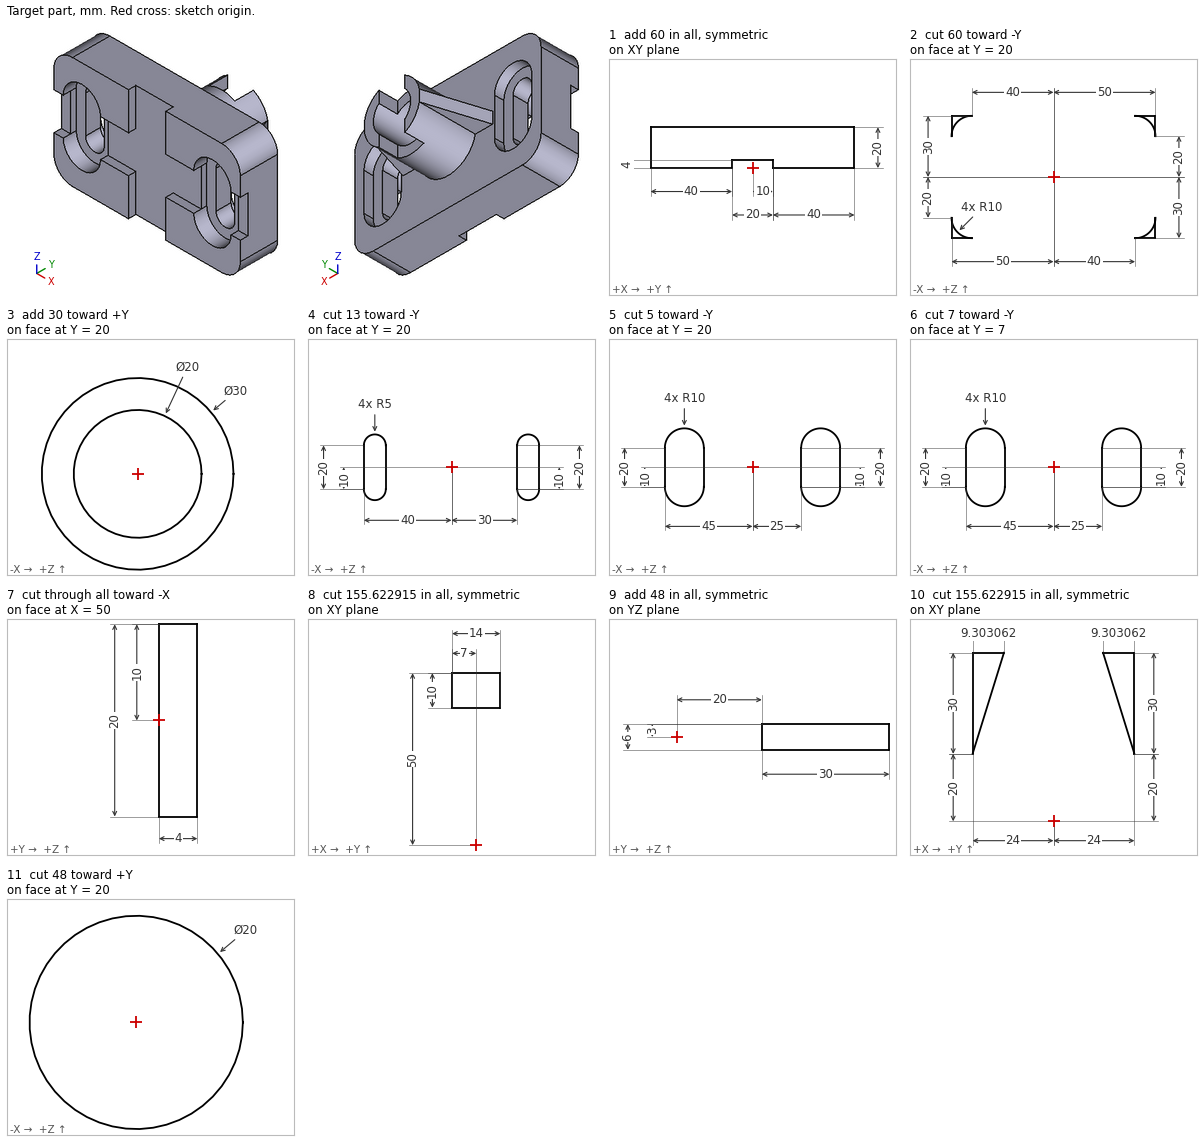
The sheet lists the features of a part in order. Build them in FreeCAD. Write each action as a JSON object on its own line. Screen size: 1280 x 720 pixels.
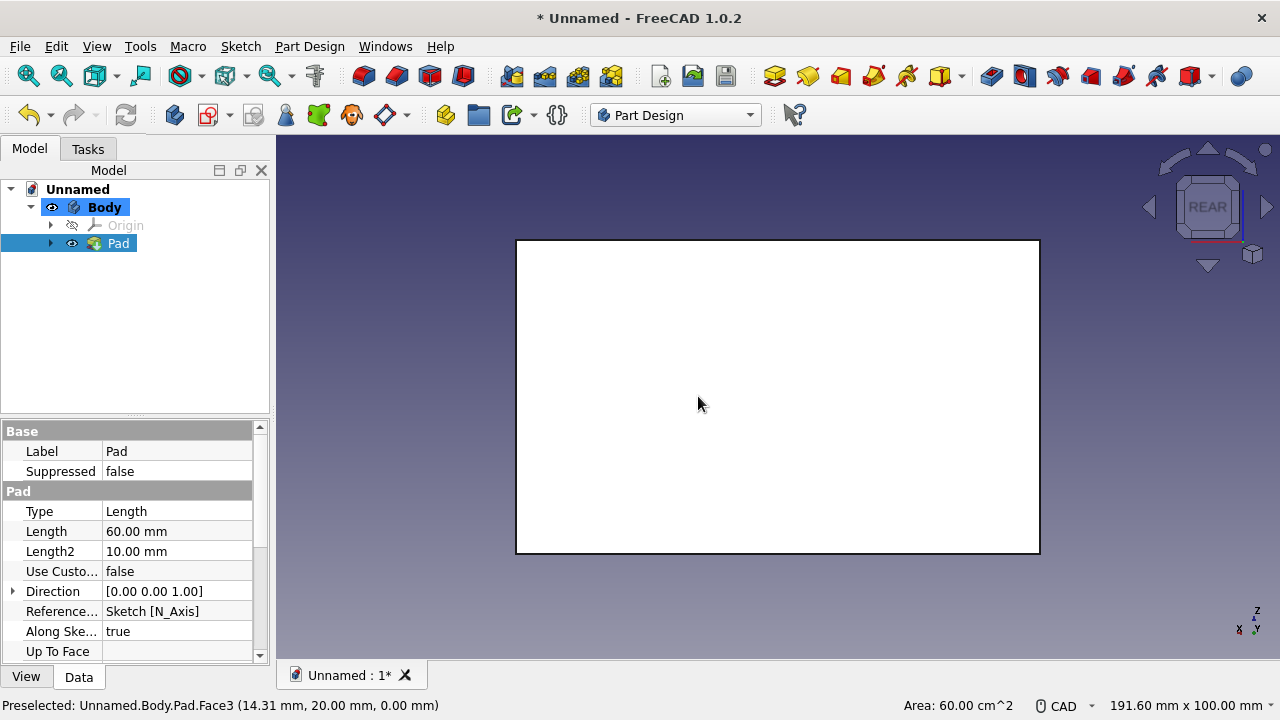
{"action": "left_click", "coordinate": [208, 116]}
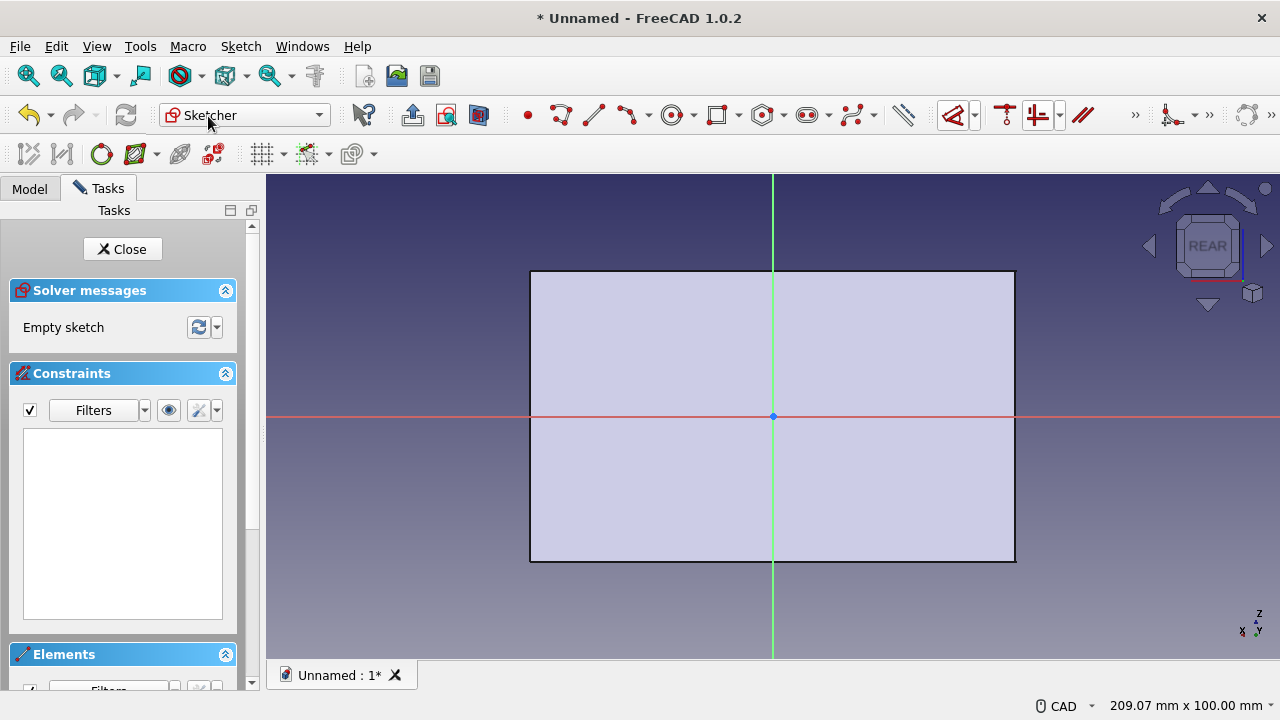
{"action": "left_click", "coordinate": [561, 116]}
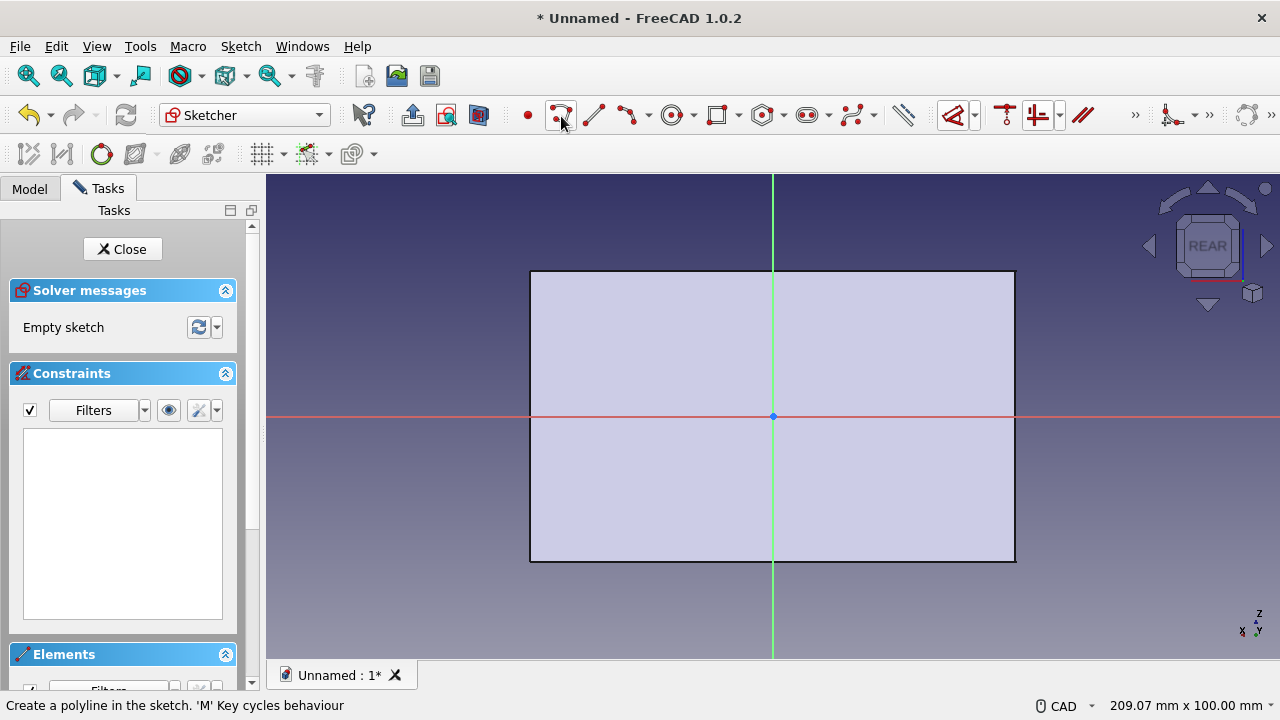
{"action": "left_click", "coordinate": [531, 513]}
{"action": "left_click", "coordinate": [531, 562]}
{"action": "left_click", "coordinate": [579, 562]}
{"action": "right_click", "coordinate": [579, 562]}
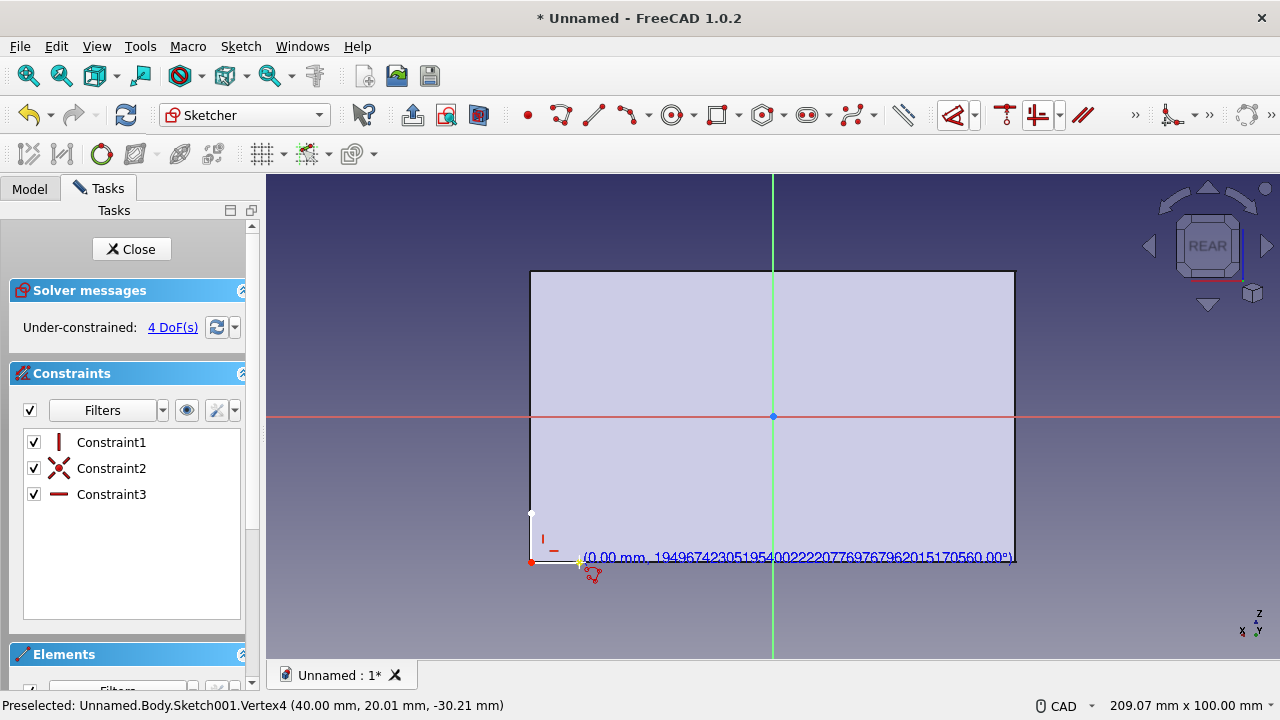
{"action": "key", "text": "g 3 a"}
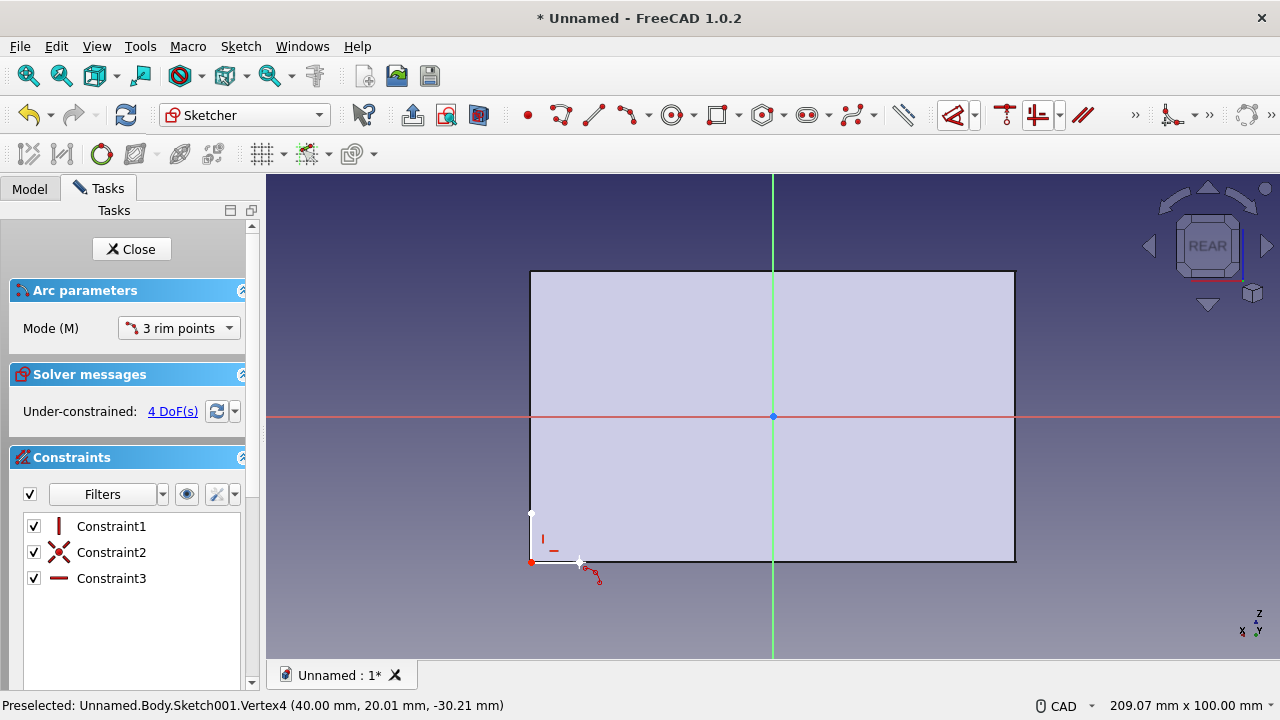
{"action": "left_click", "coordinate": [579, 563]}
{"action": "left_click", "coordinate": [531, 514]}
{"action": "left_click", "coordinate": [545, 548]}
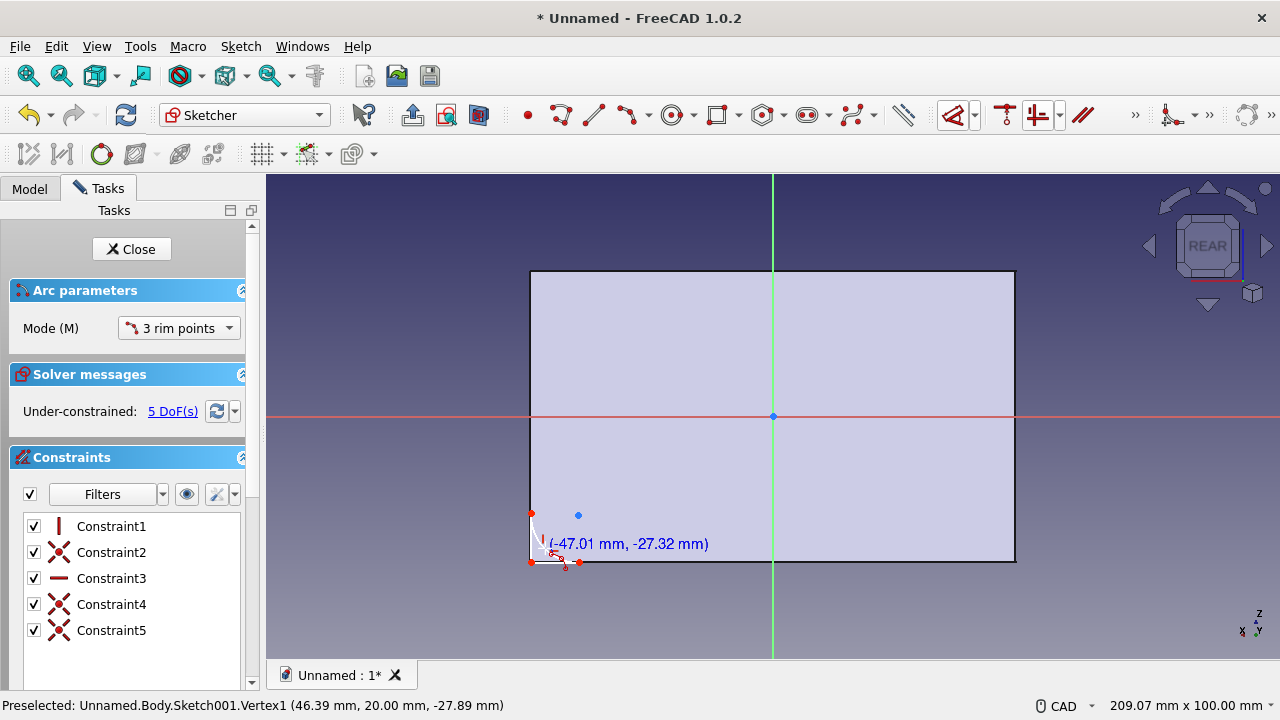
{"action": "key", "text": "g m"}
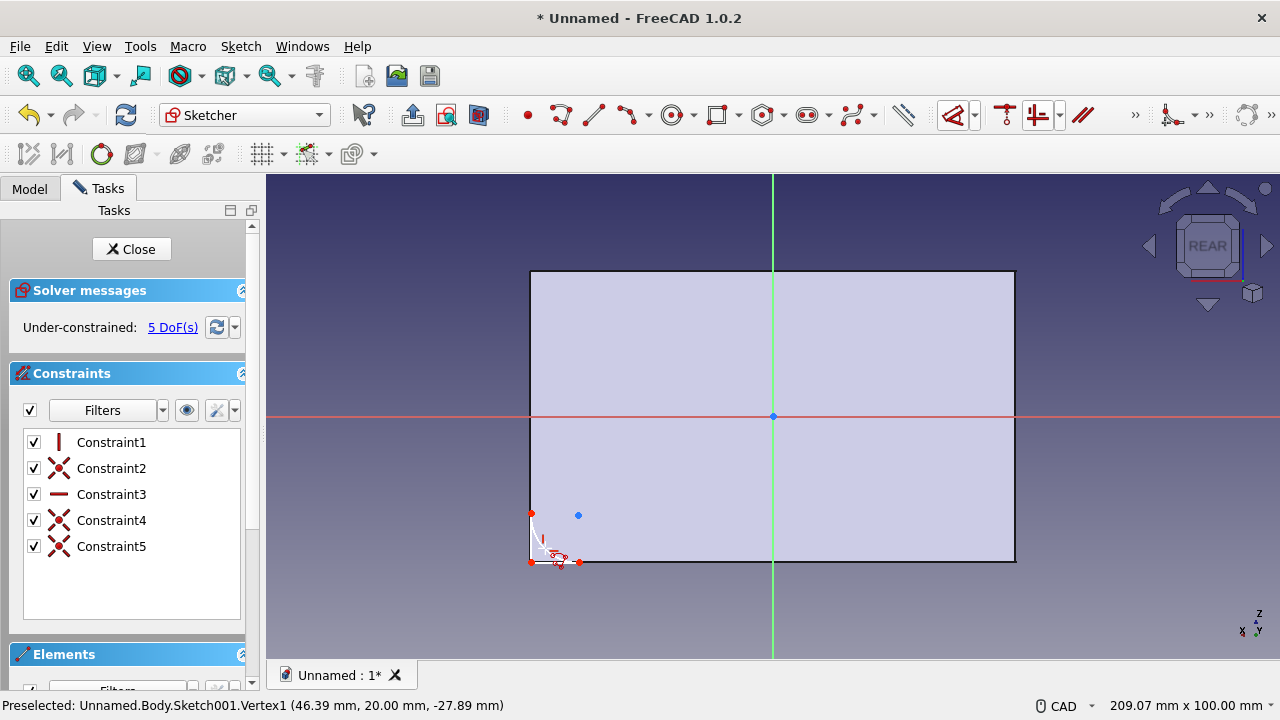
{"action": "left_click", "coordinate": [967, 562]}
{"action": "left_click", "coordinate": [1016, 562]}
{"action": "left_click", "coordinate": [1016, 513]}
{"action": "right_click", "coordinate": [1016, 513]}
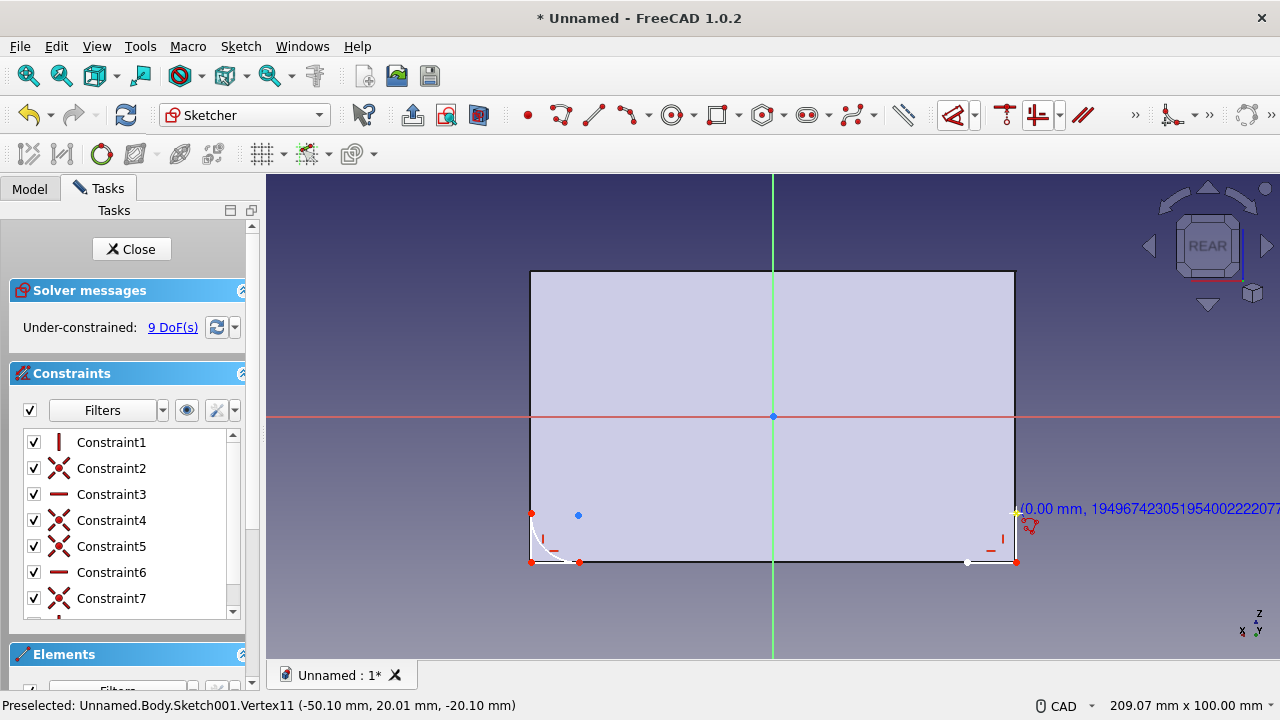
{"action": "key", "text": "g 3 a"}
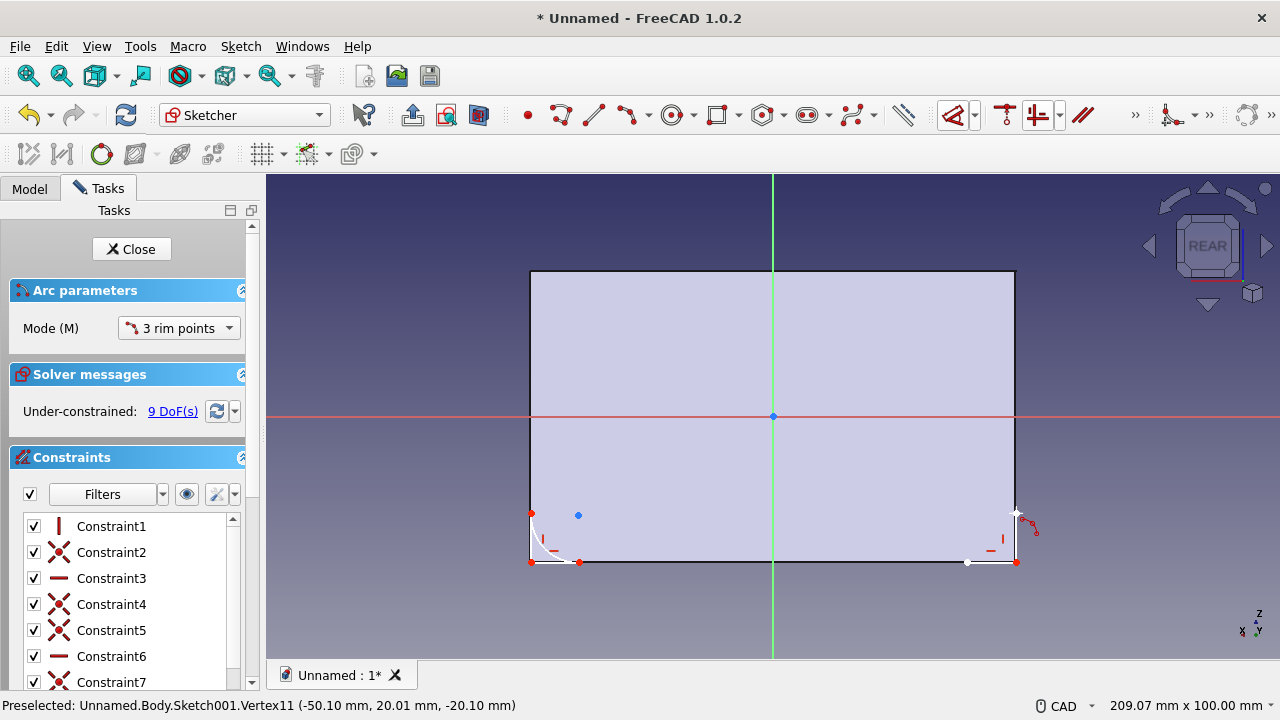
{"action": "left_click", "coordinate": [1016, 514]}
{"action": "left_click", "coordinate": [967, 563]}
{"action": "left_click", "coordinate": [1001, 548]}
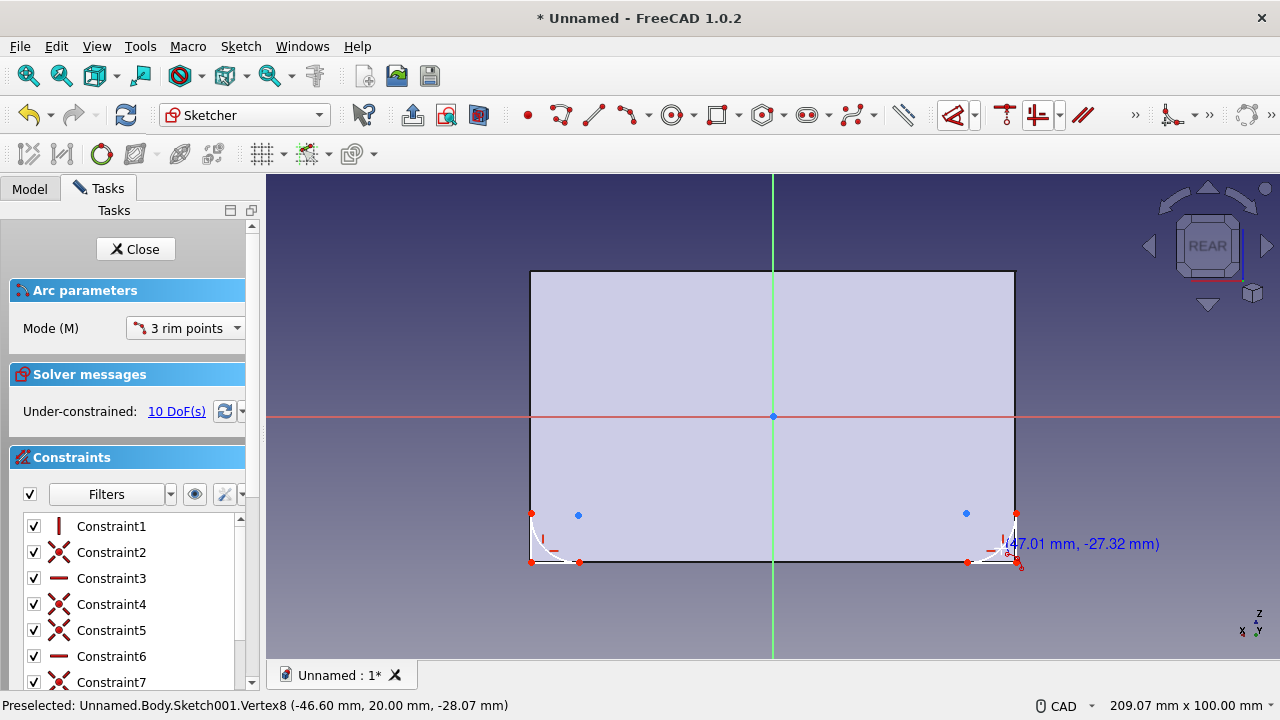
{"action": "key", "text": "g m"}